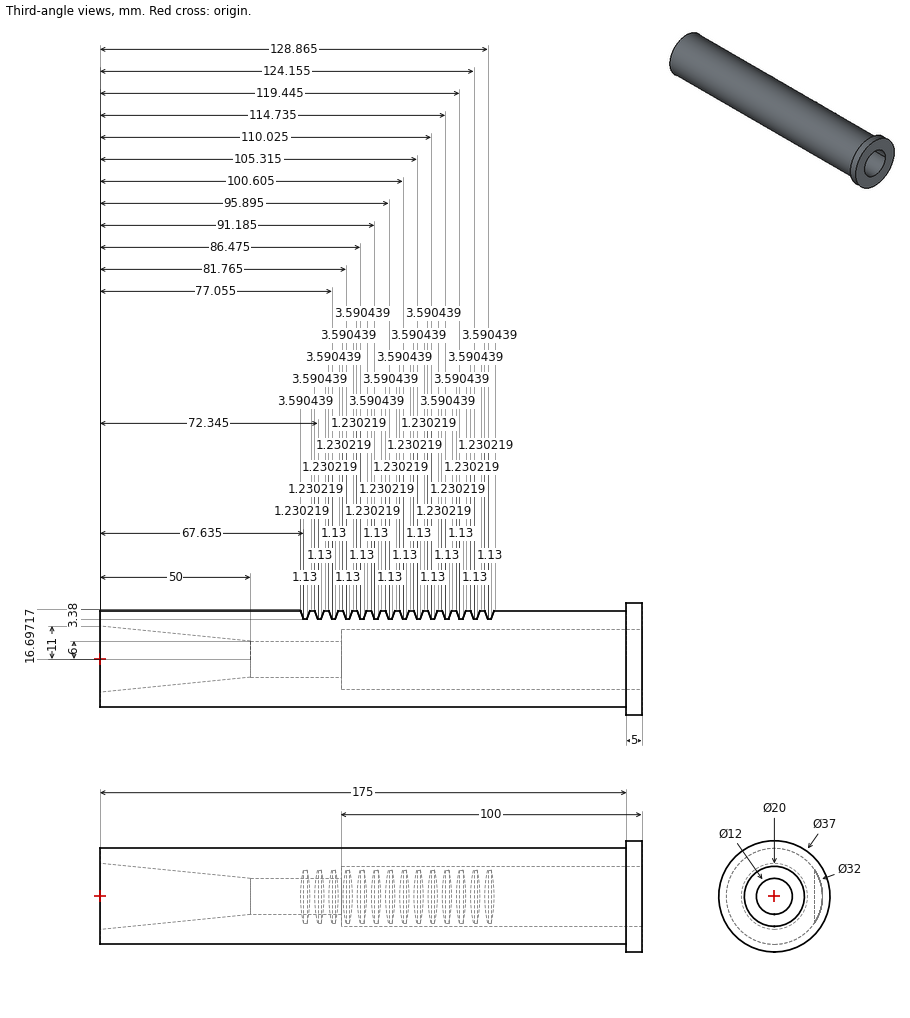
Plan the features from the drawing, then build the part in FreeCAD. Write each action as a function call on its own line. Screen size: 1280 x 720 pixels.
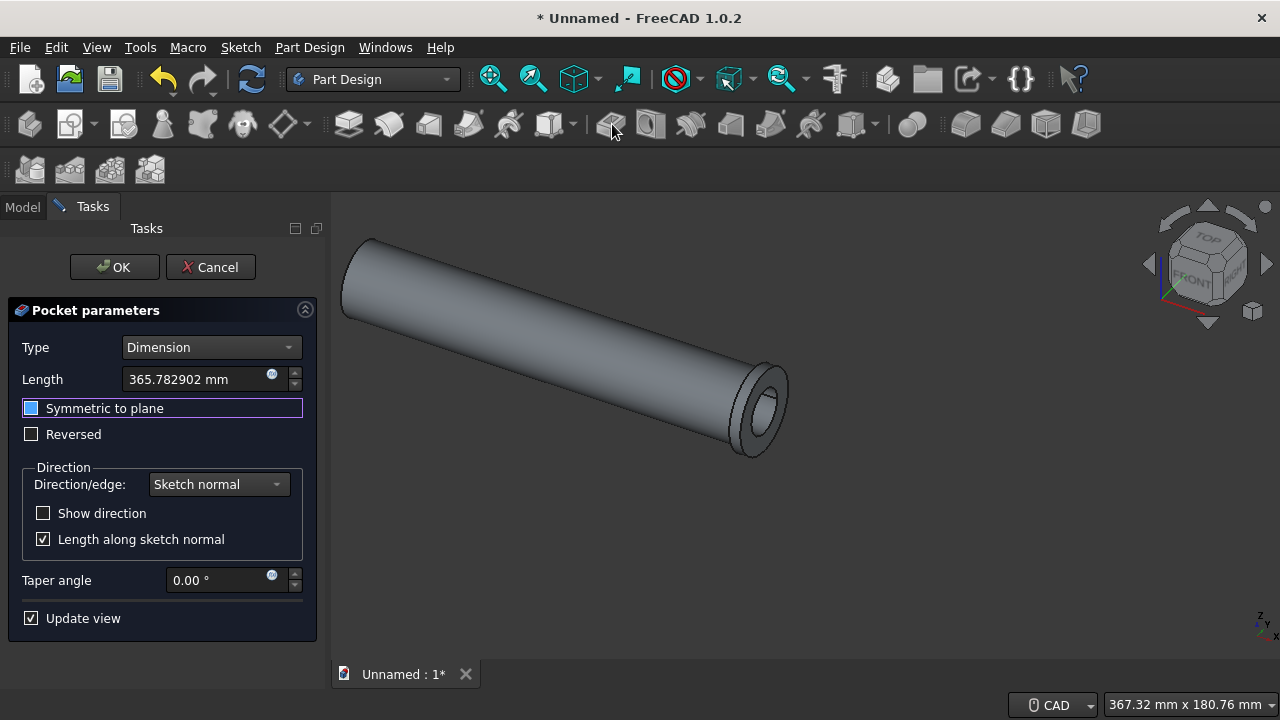
click(30, 408)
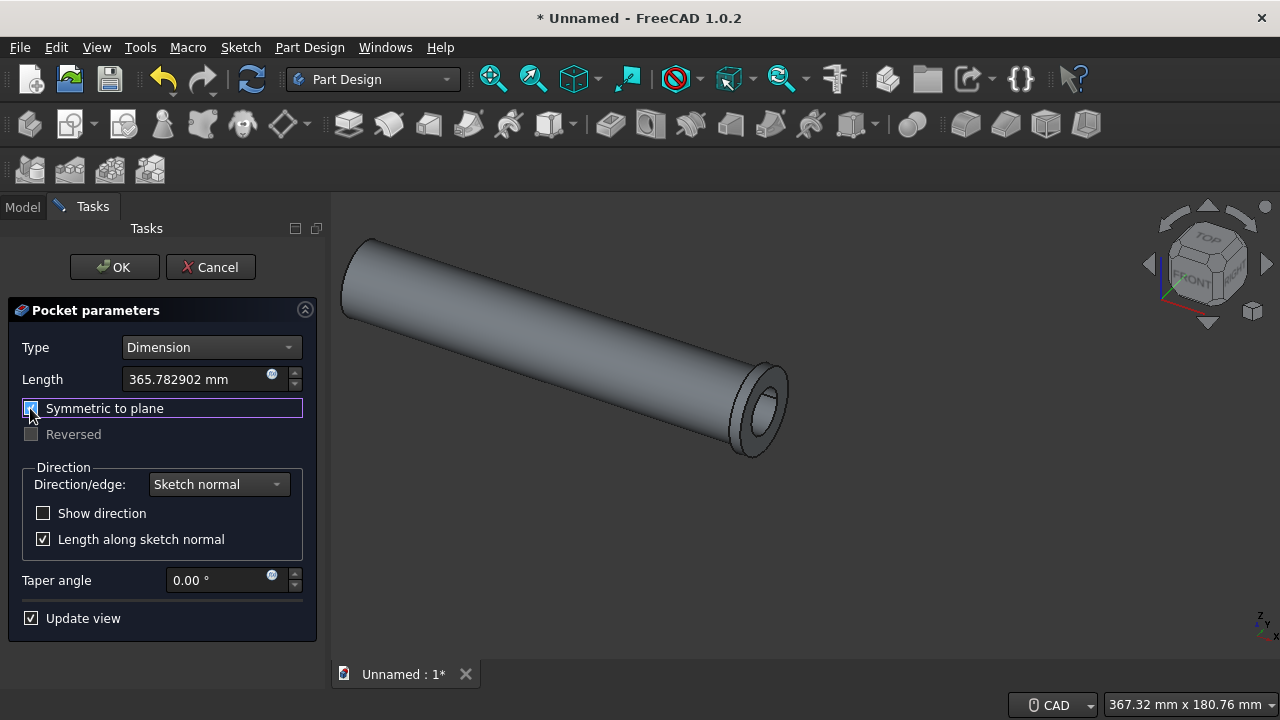
click(115, 267)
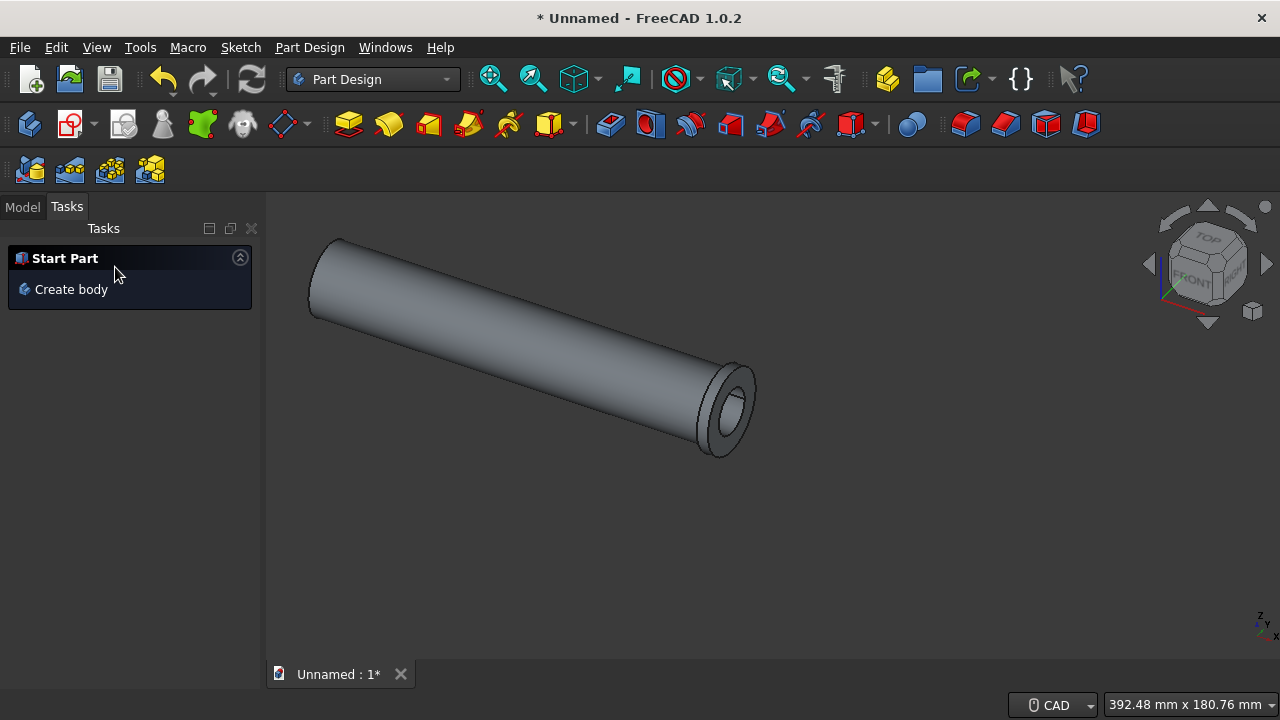
key(0)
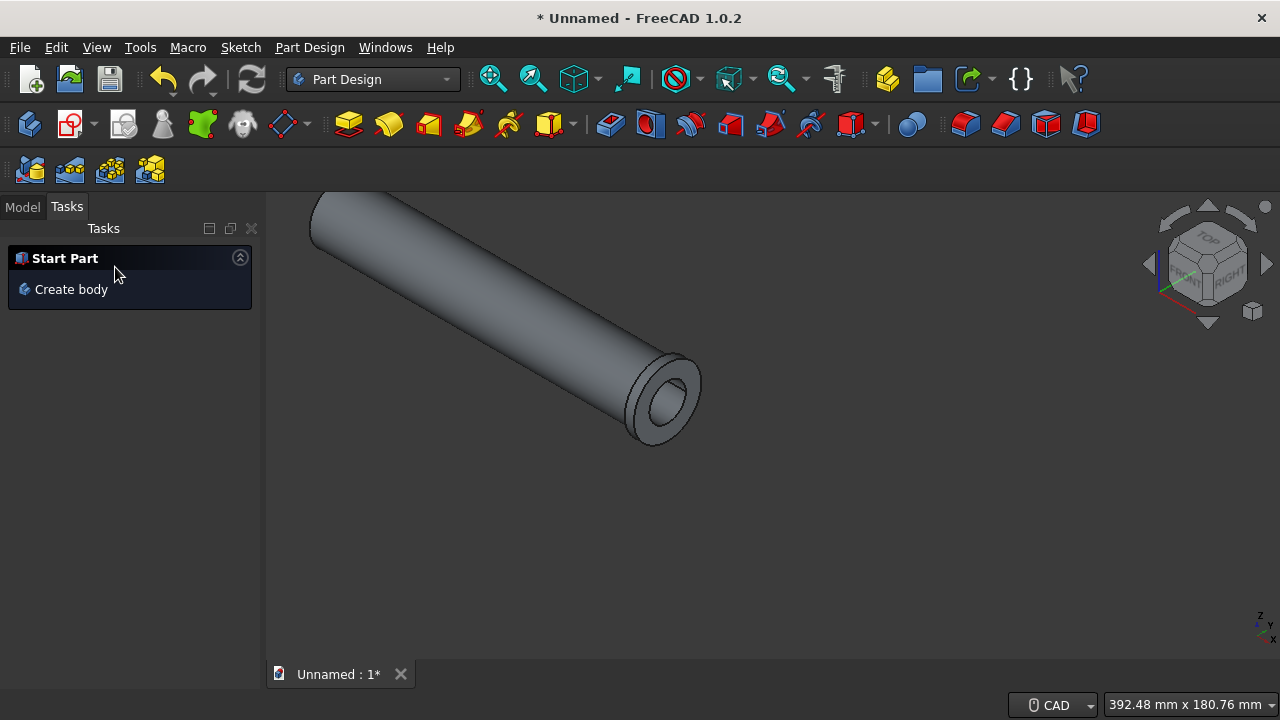
click(494, 80)